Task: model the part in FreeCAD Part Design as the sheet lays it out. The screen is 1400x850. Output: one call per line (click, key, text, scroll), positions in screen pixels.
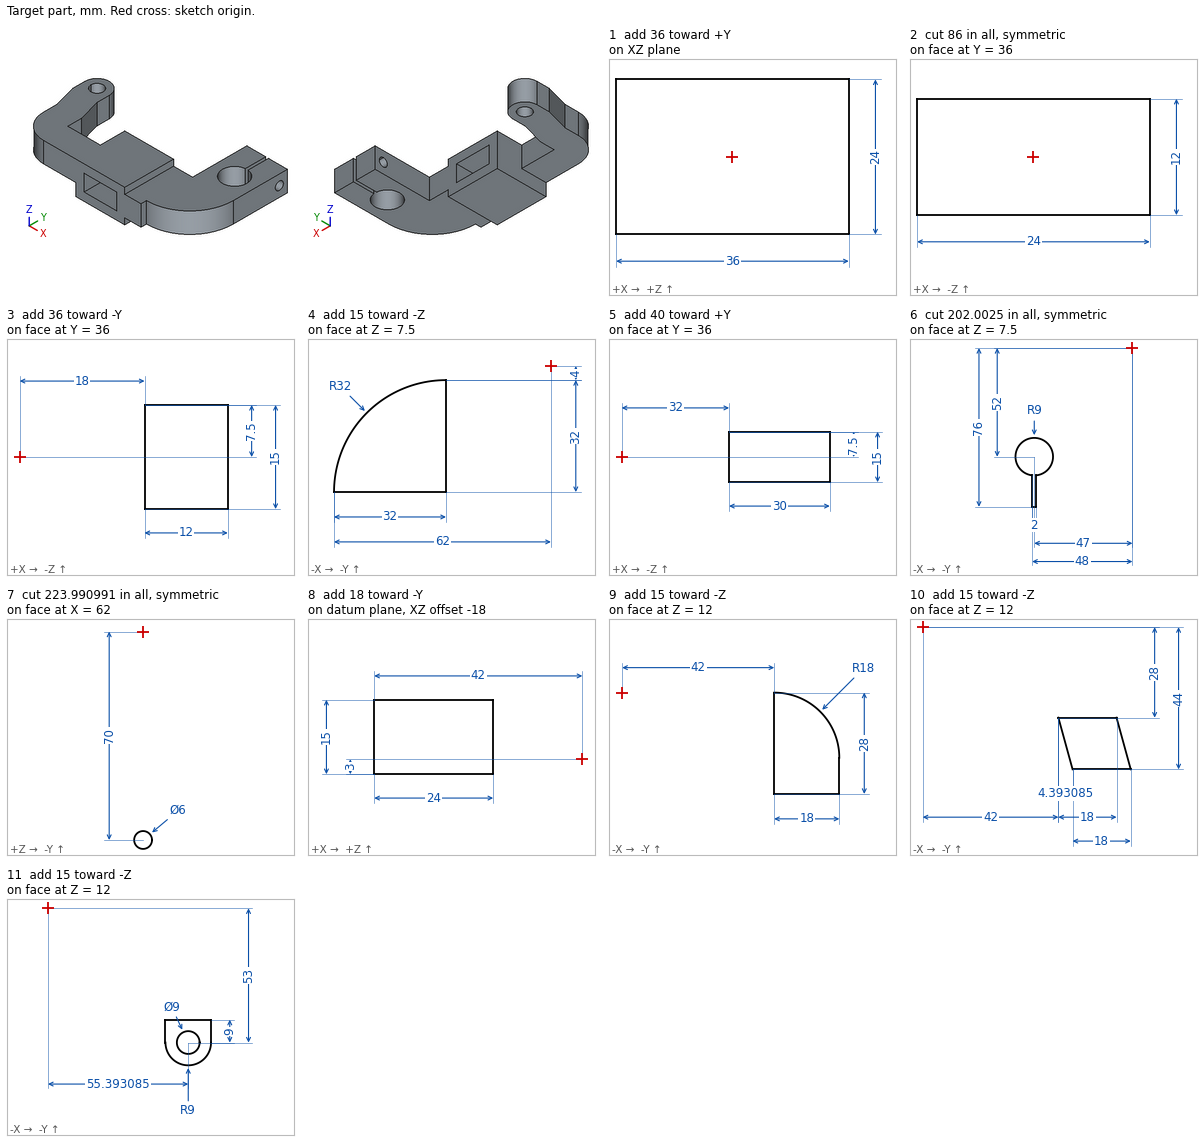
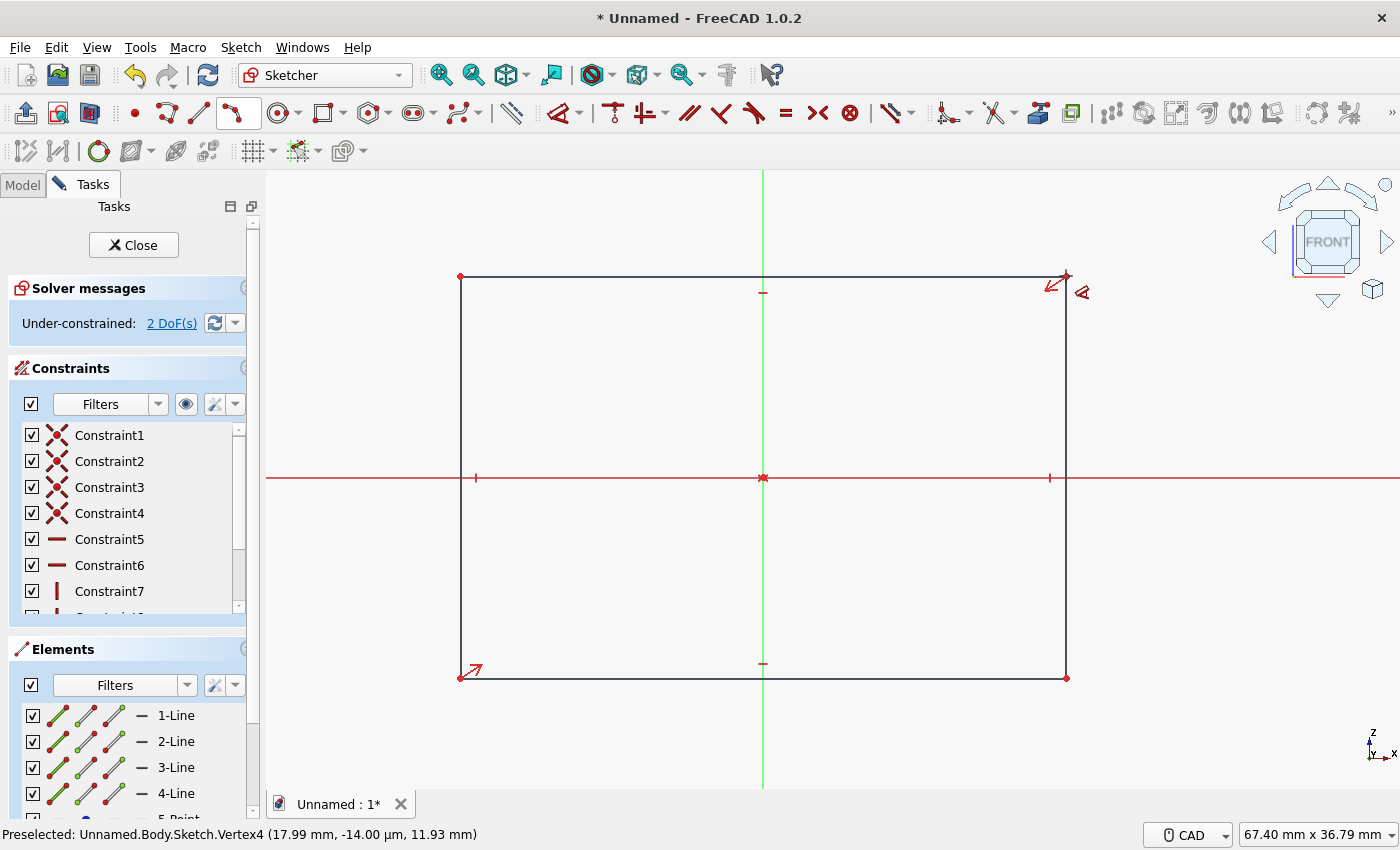
click(642, 679)
click(624, 713)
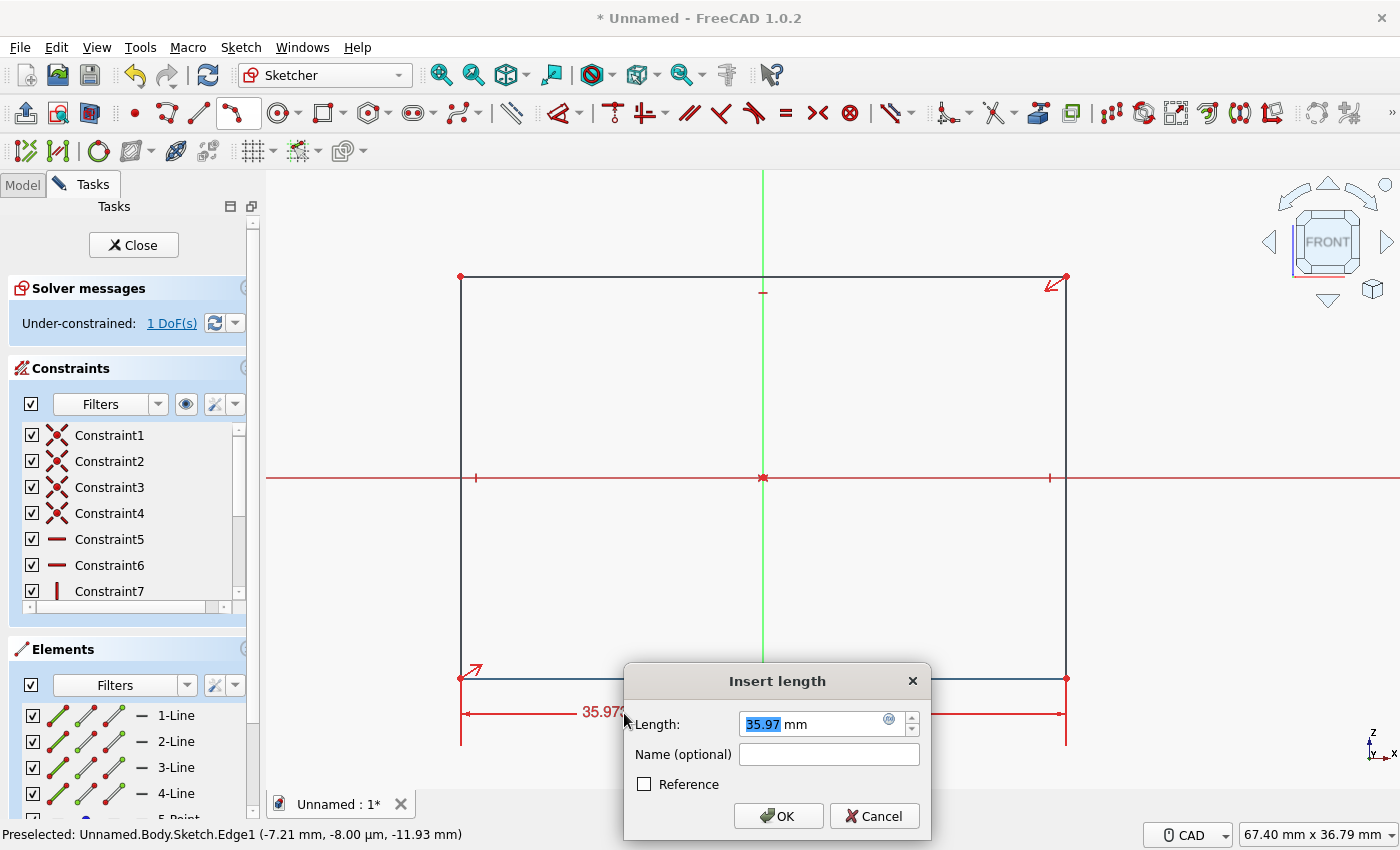
text(36)
key(Return)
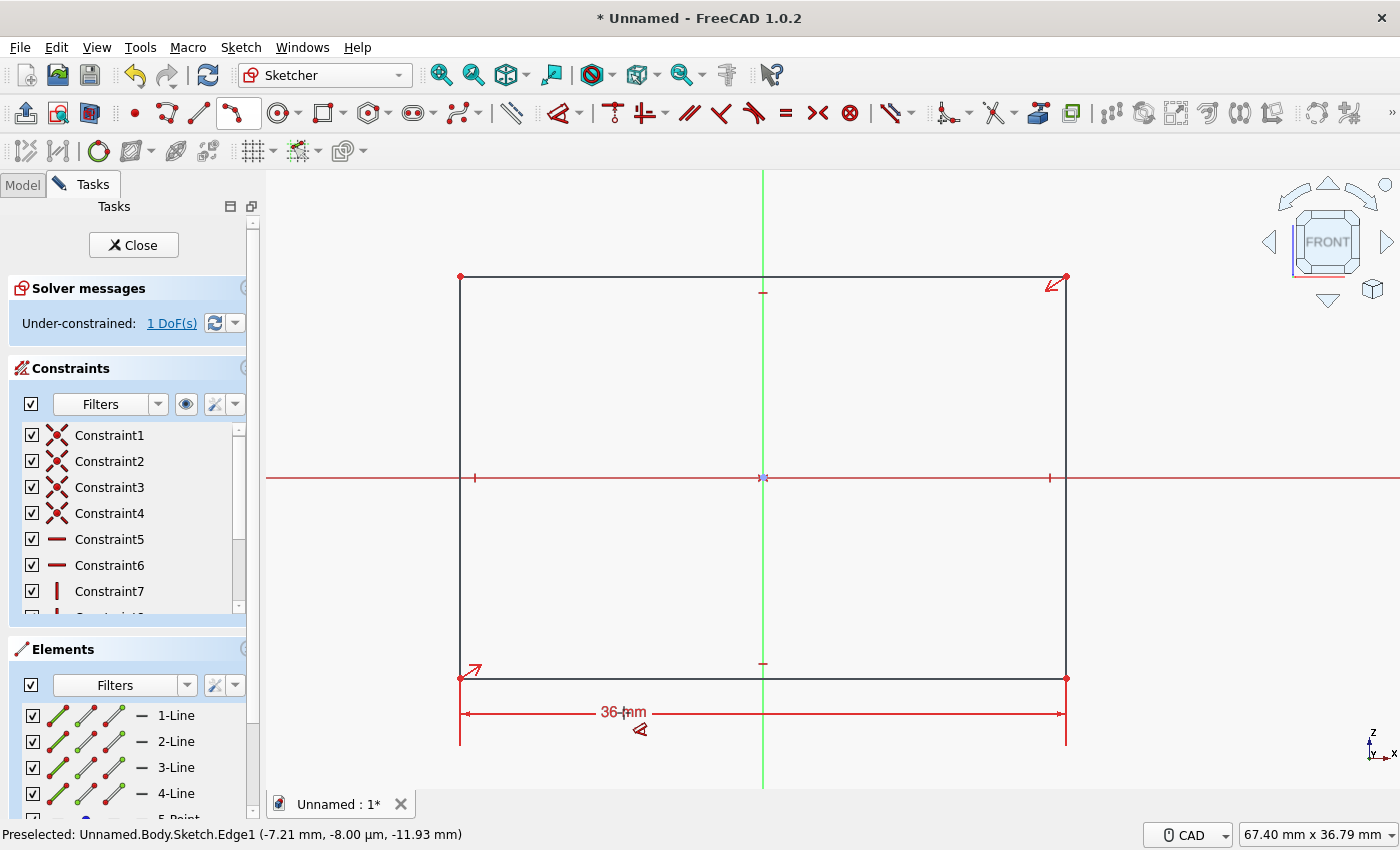
click(1066, 558)
click(1100, 385)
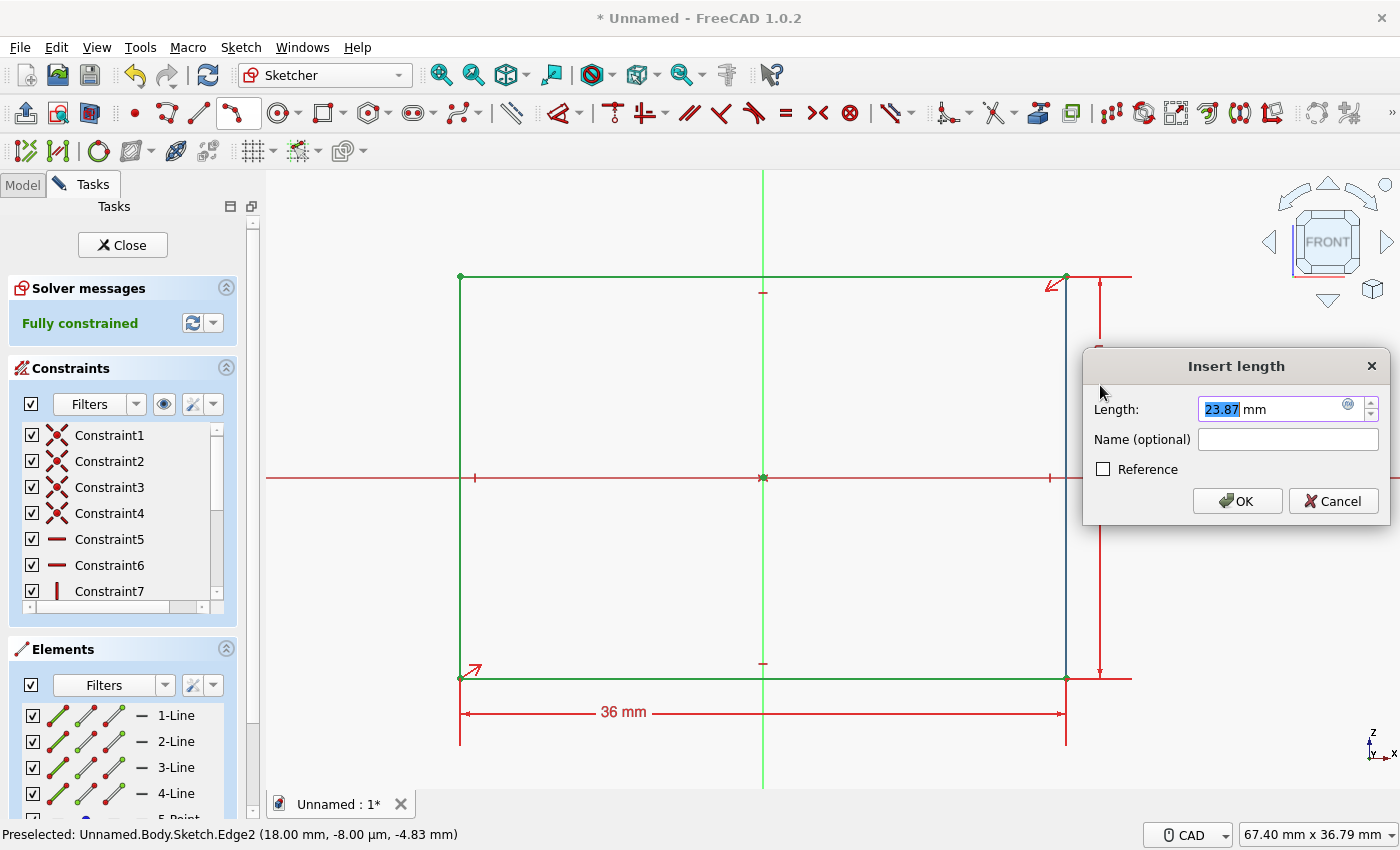
text(24)
key(Return)
key(Escape)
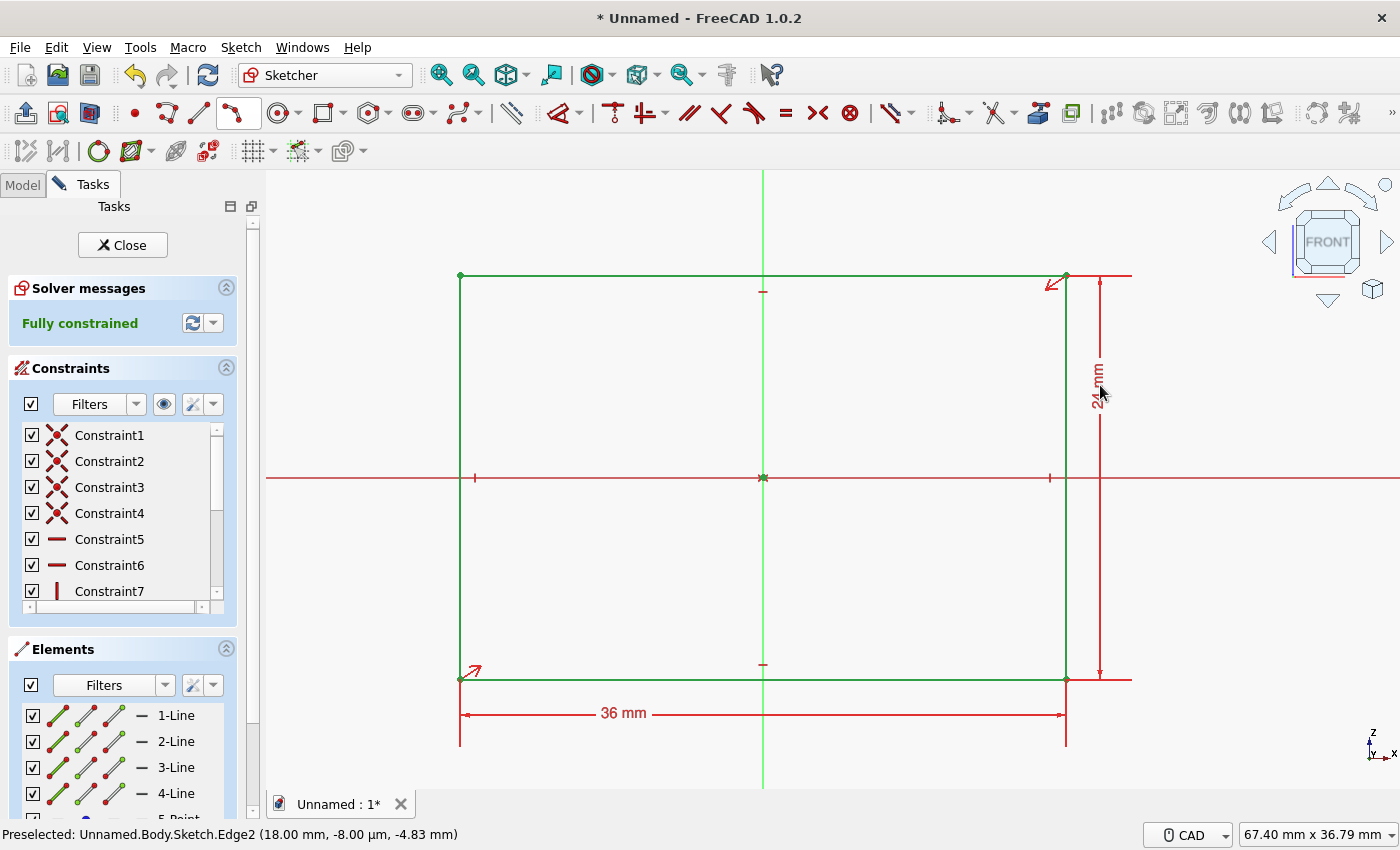
click(123, 245)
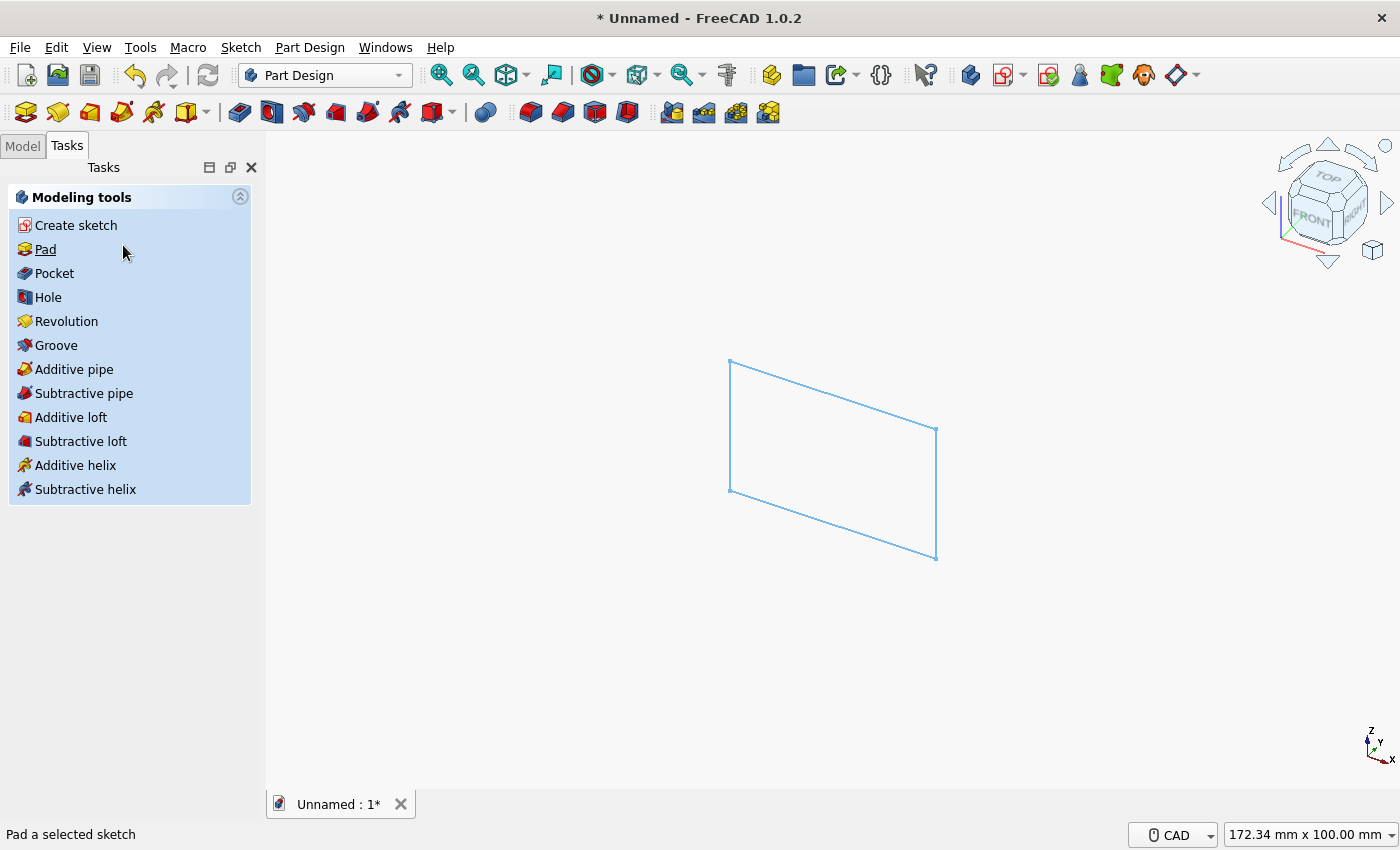
click(26, 112)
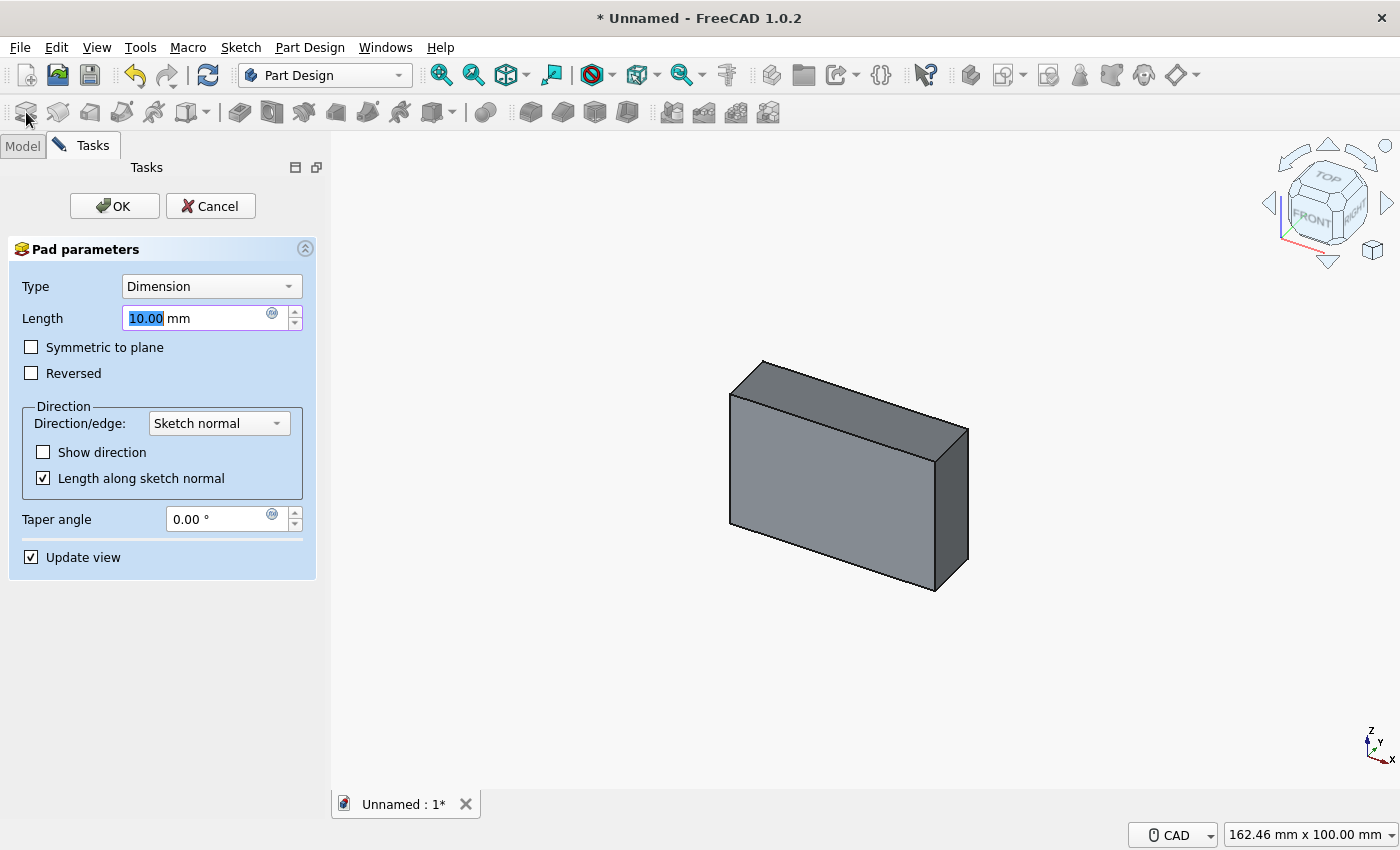
text(36)
key(Tab)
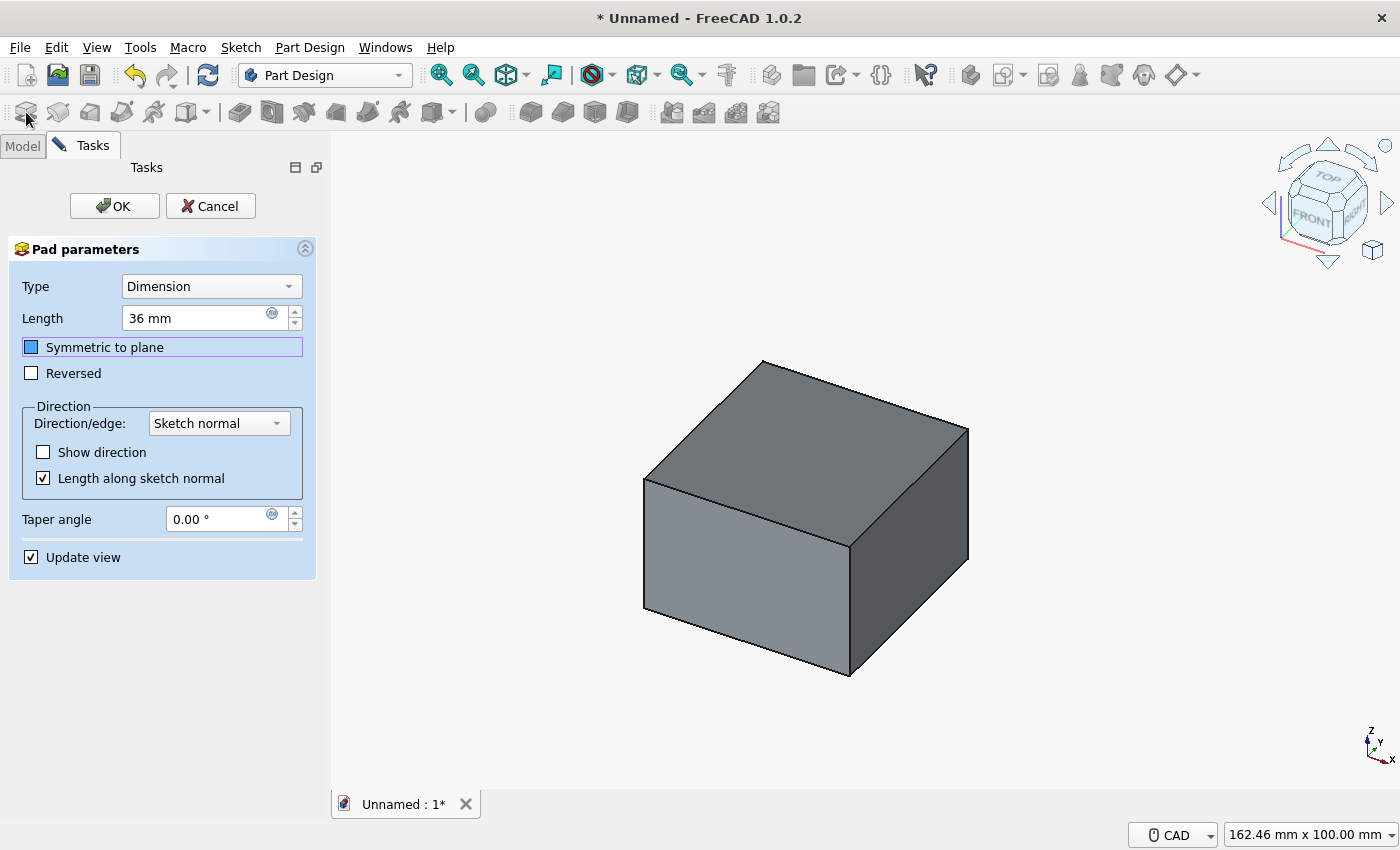
click(30, 373)